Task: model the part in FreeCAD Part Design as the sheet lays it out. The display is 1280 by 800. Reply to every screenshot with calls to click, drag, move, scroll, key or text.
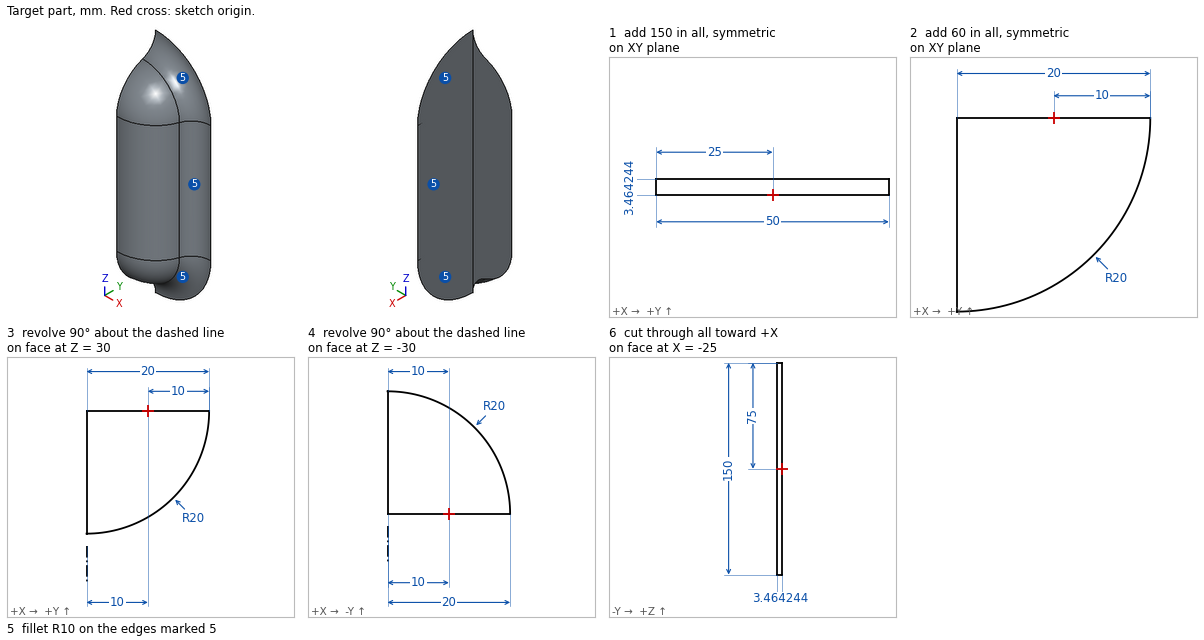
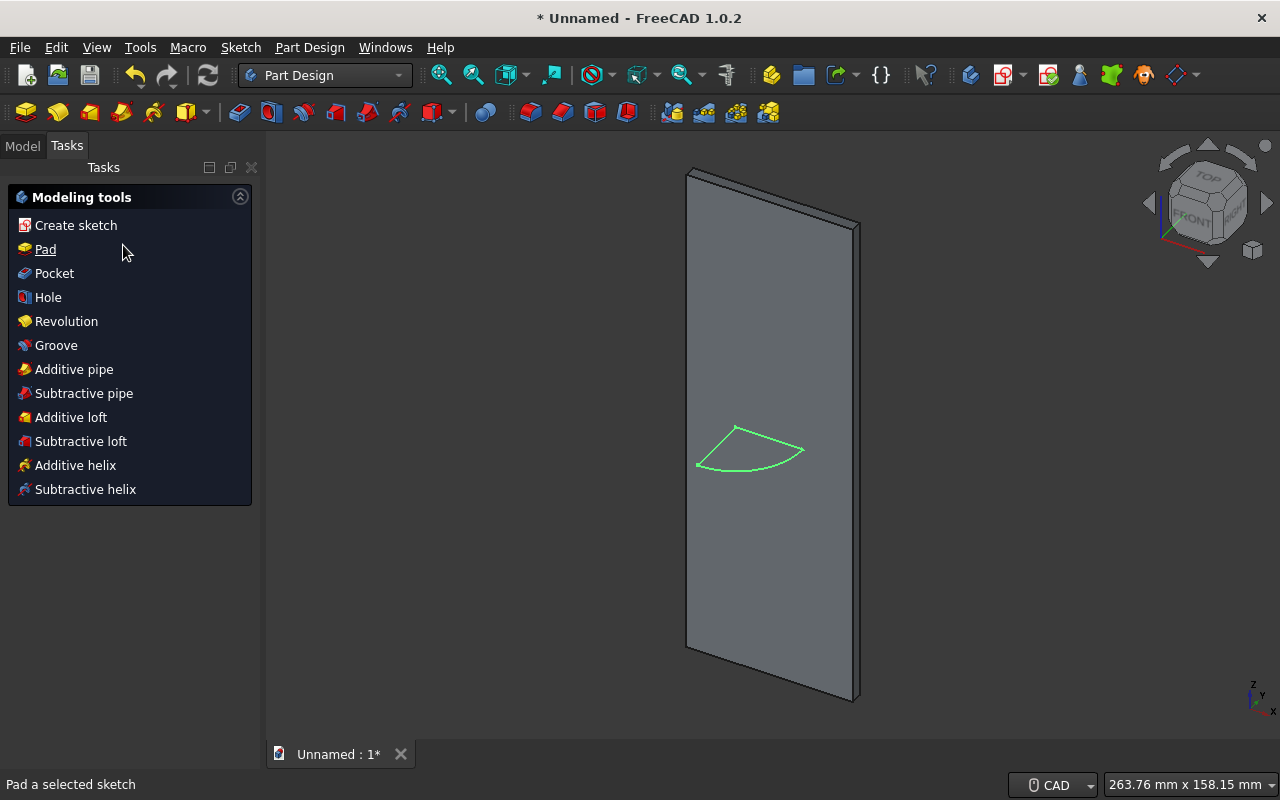
click(26, 112)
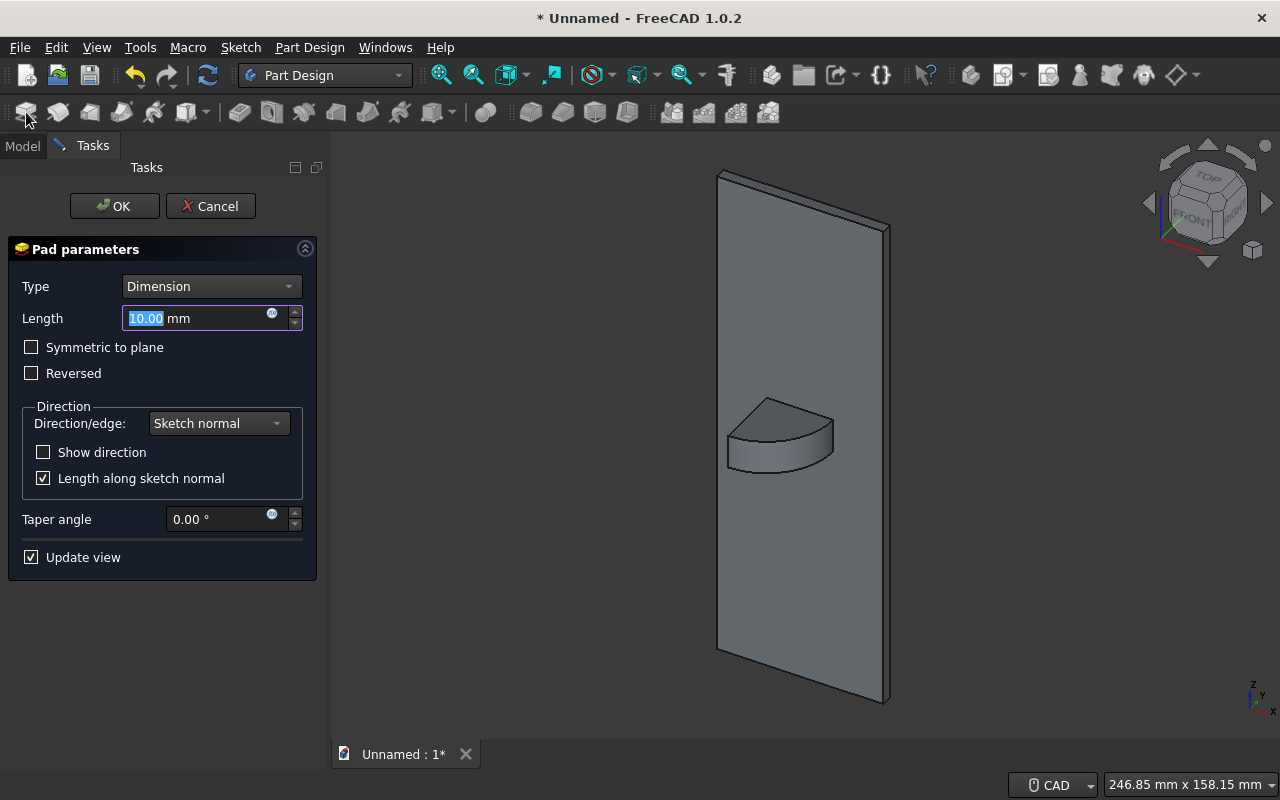
text(60)
key(Tab)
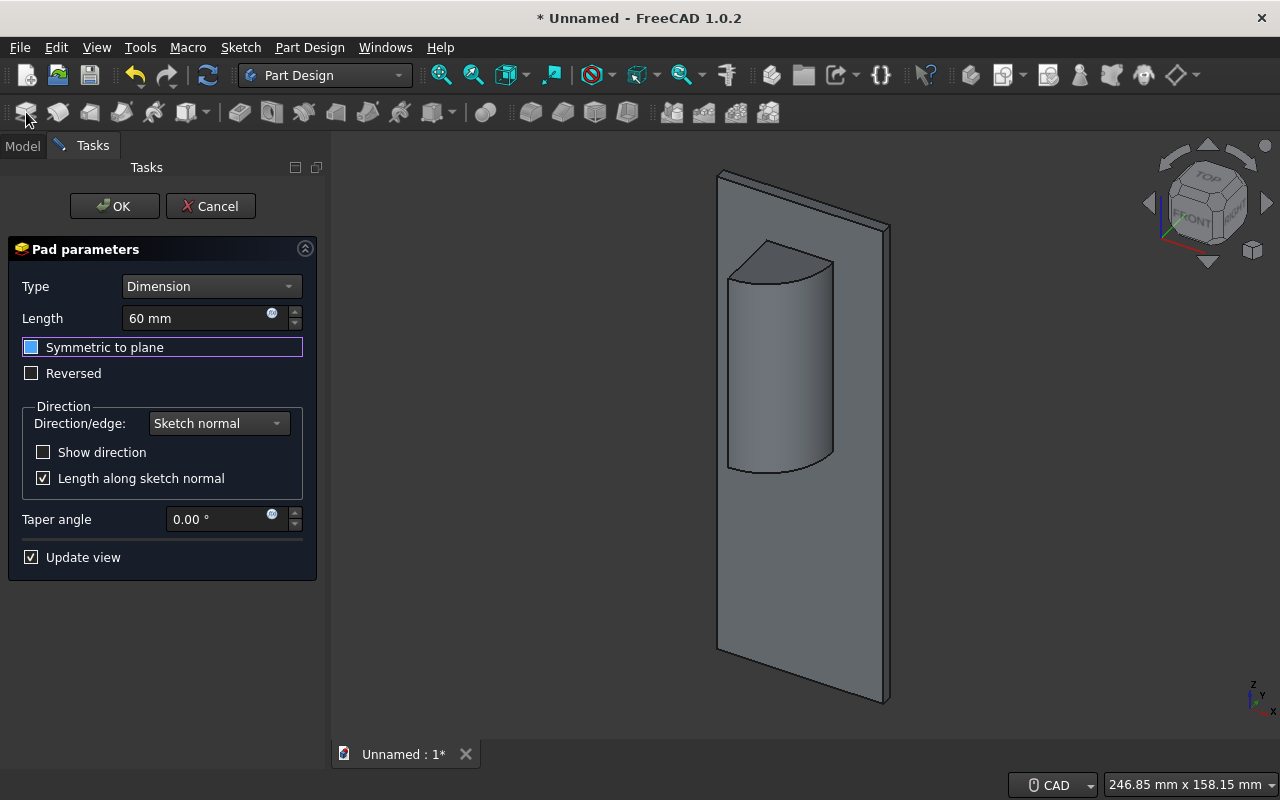
click(30, 347)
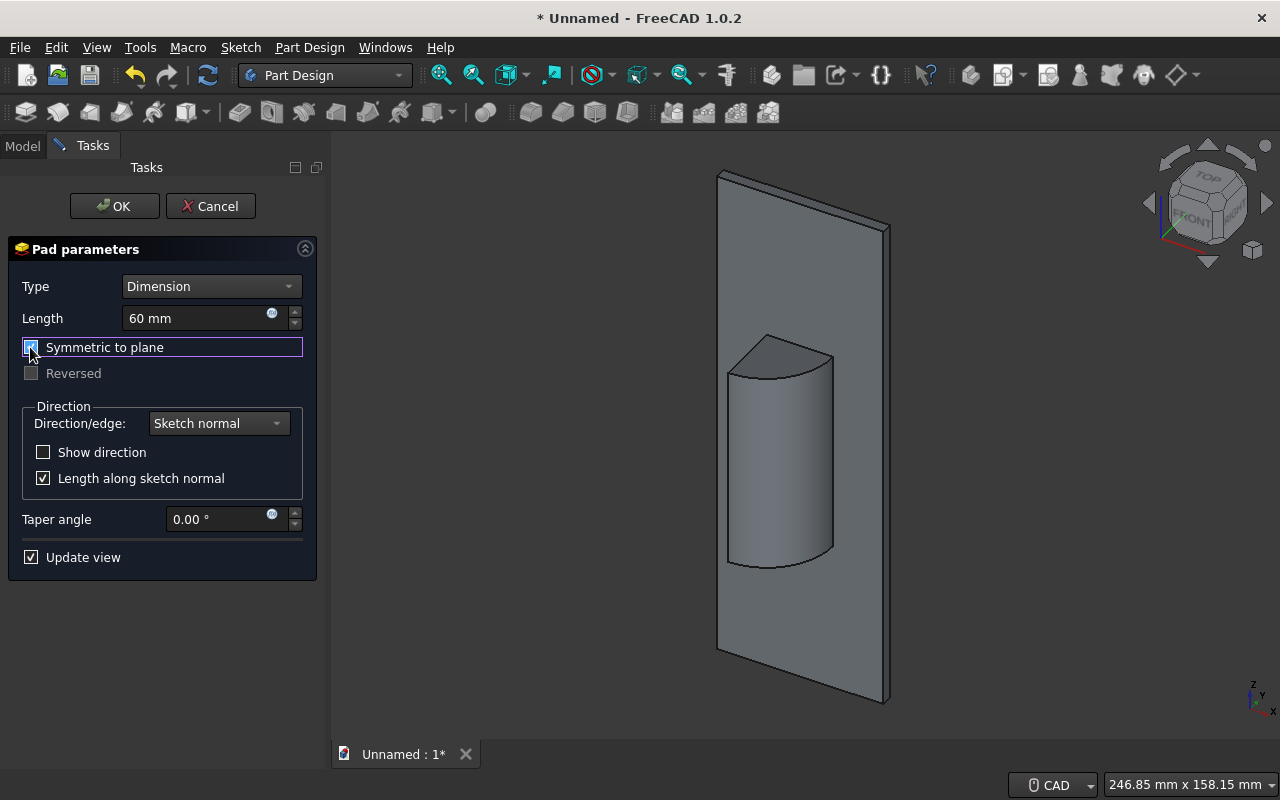
click(115, 206)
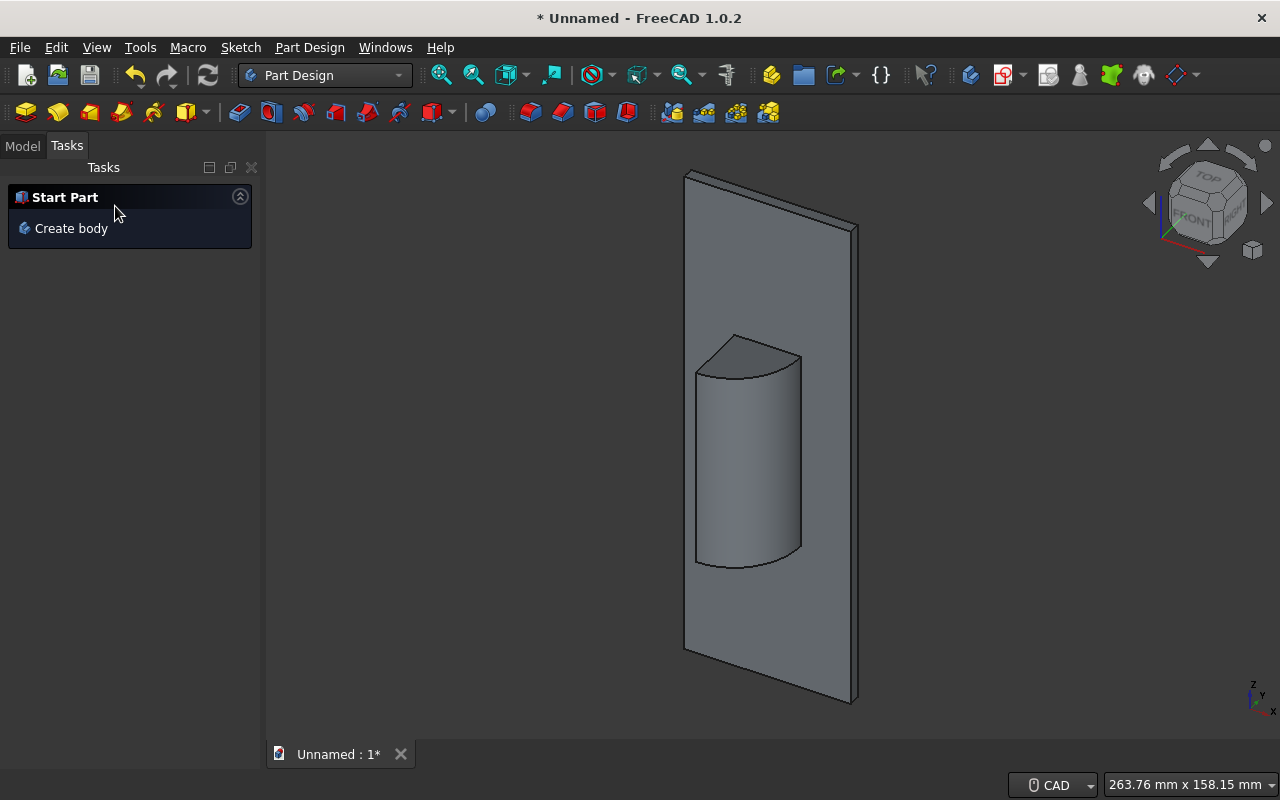
click(442, 76)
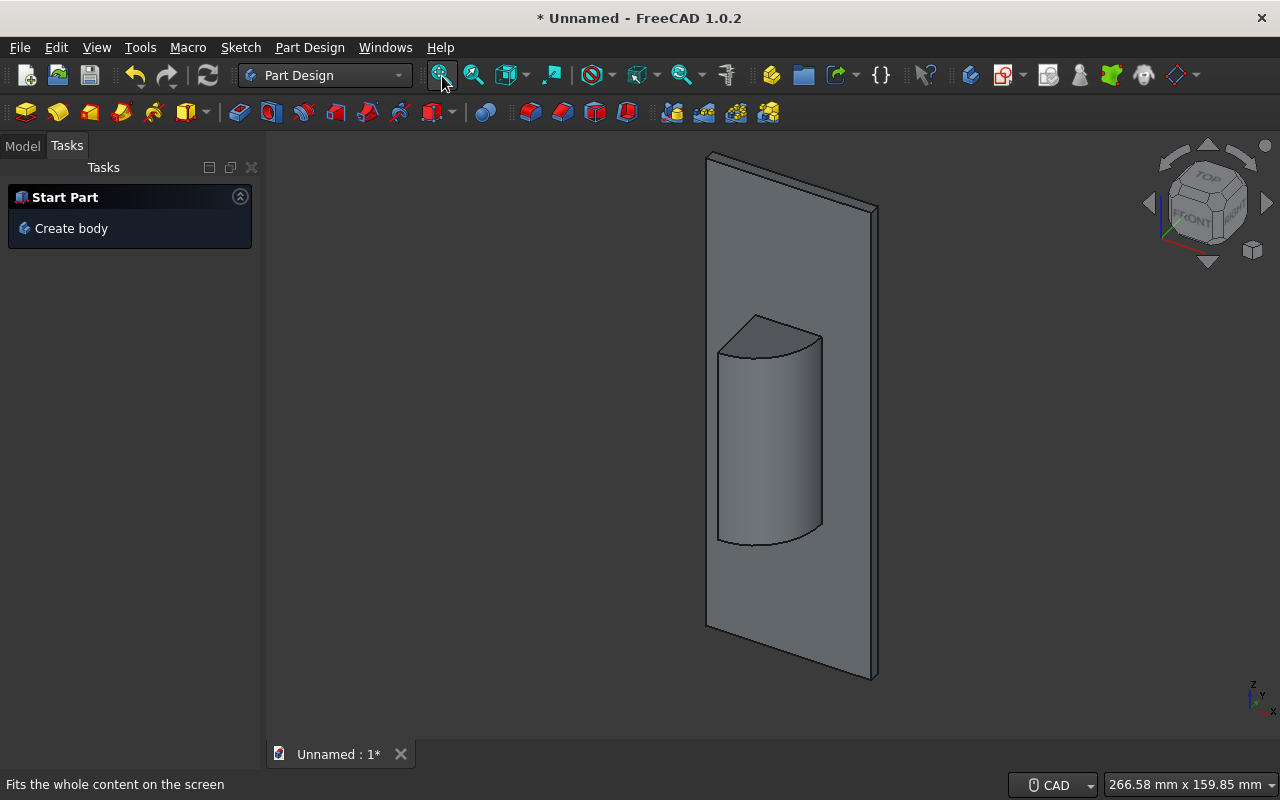
click(760, 341)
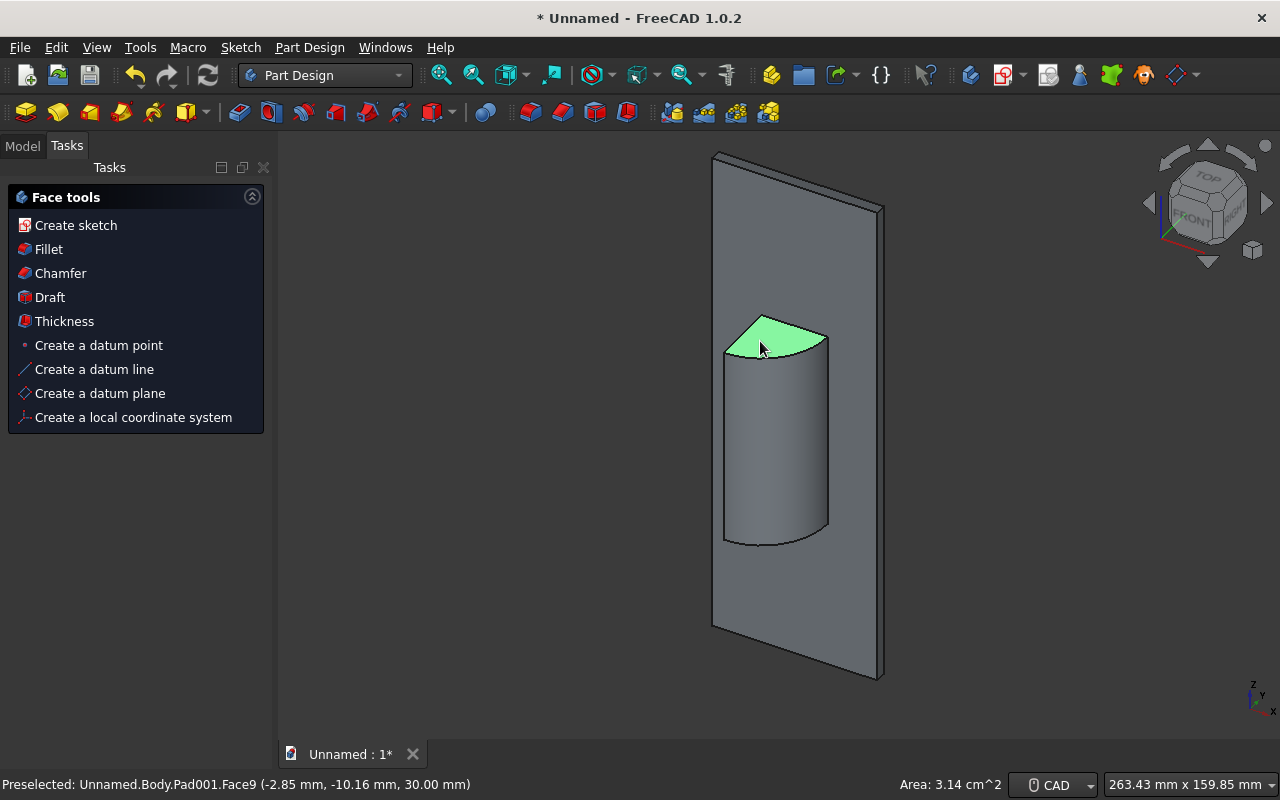
click(1004, 76)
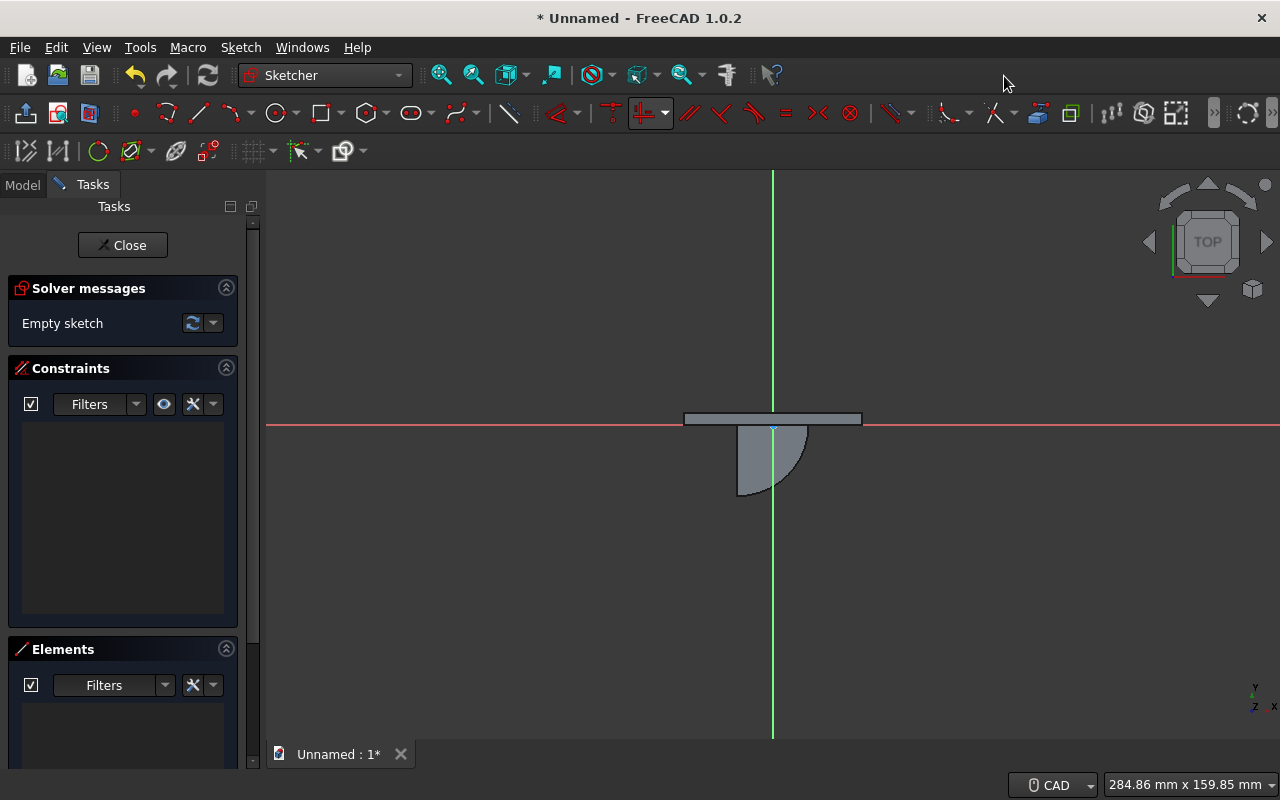
scroll(803, 484, up, 6)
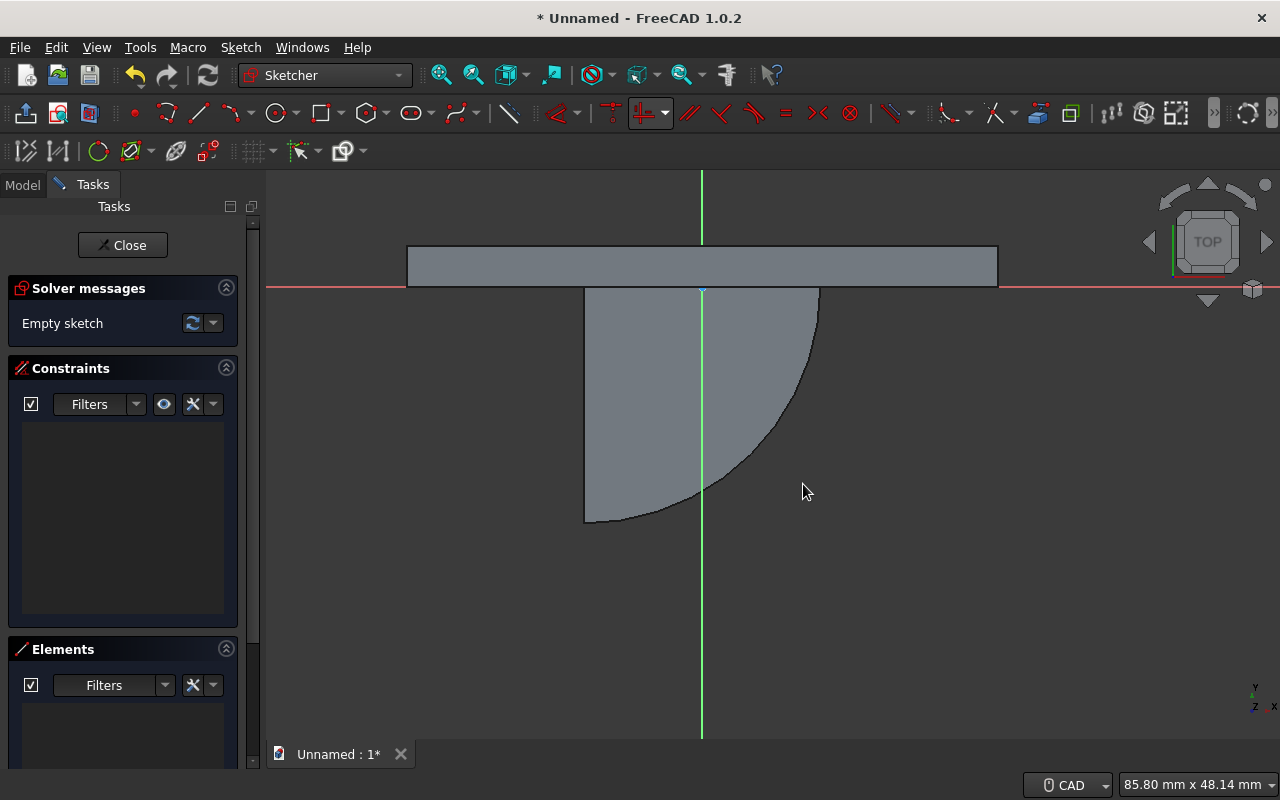
click(168, 114)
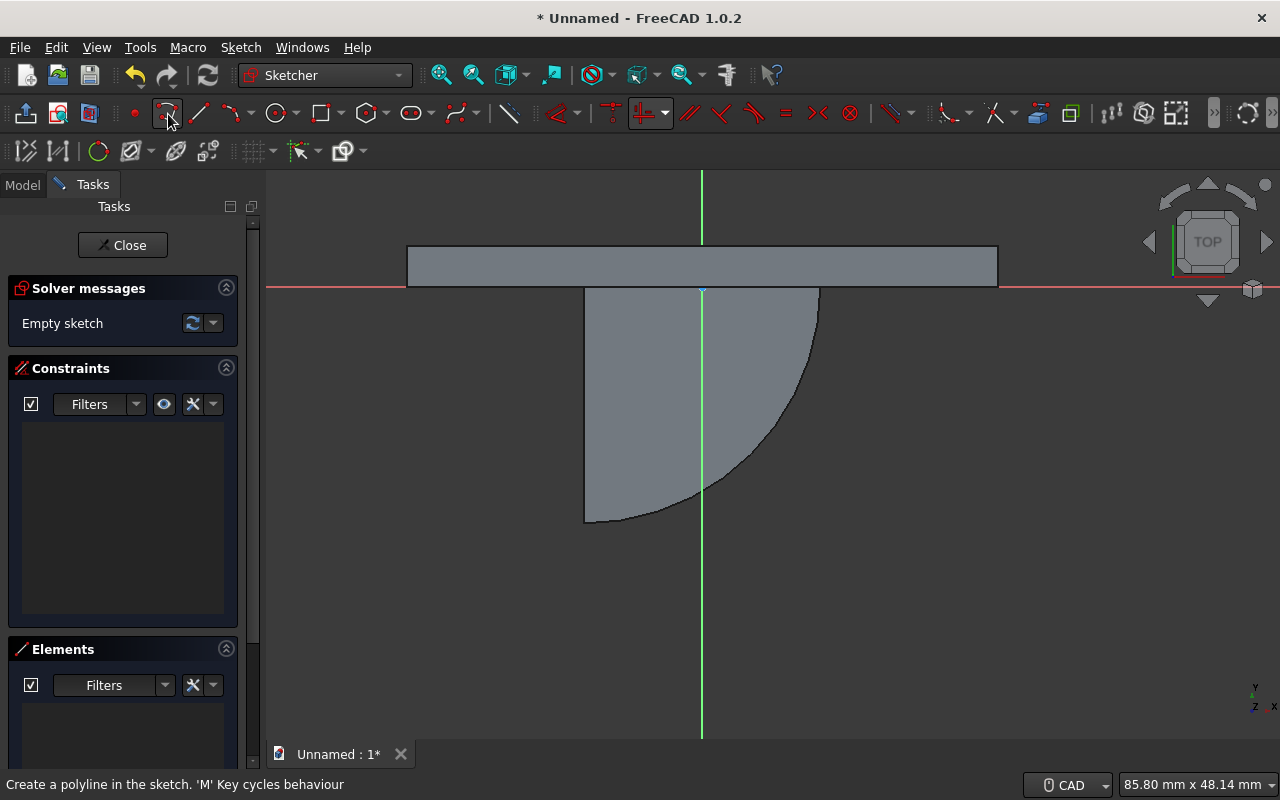
click(820, 287)
click(584, 296)
click(584, 523)
right_click(584, 523)